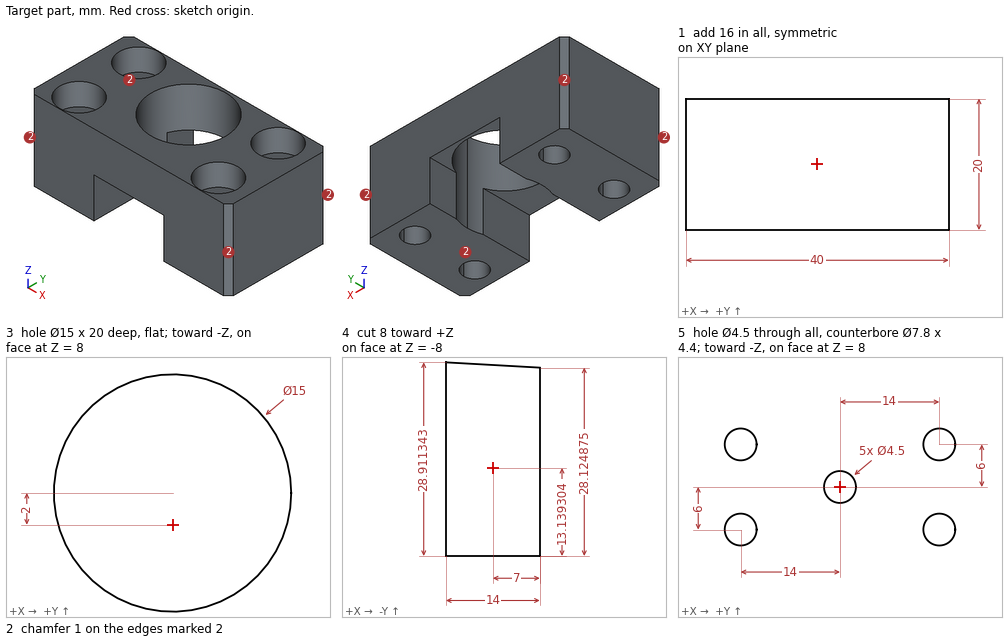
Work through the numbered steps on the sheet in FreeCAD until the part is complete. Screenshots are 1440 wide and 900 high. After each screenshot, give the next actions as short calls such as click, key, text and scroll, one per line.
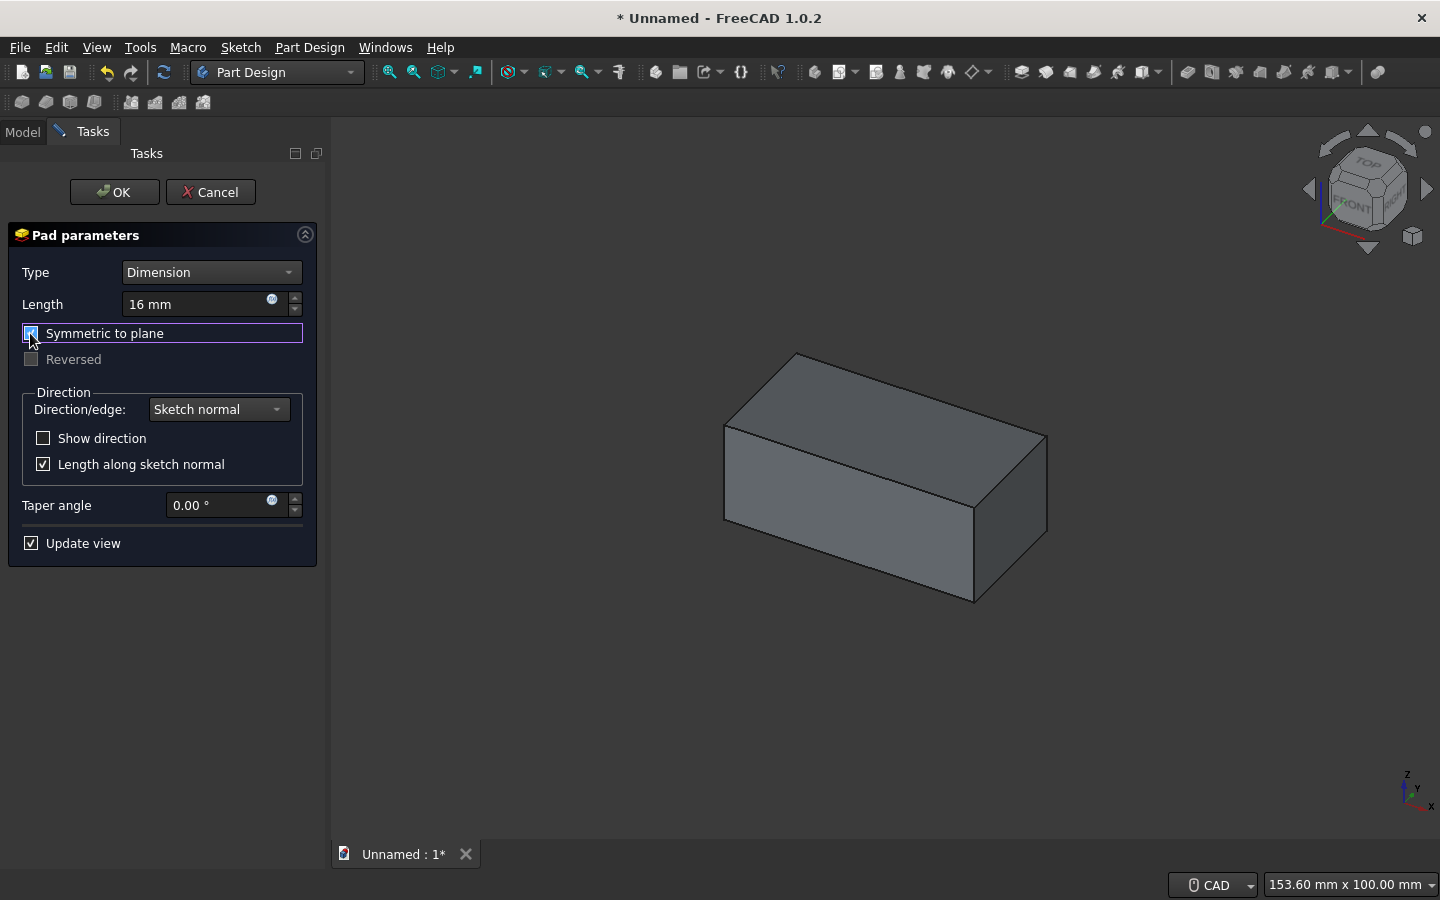
click(115, 192)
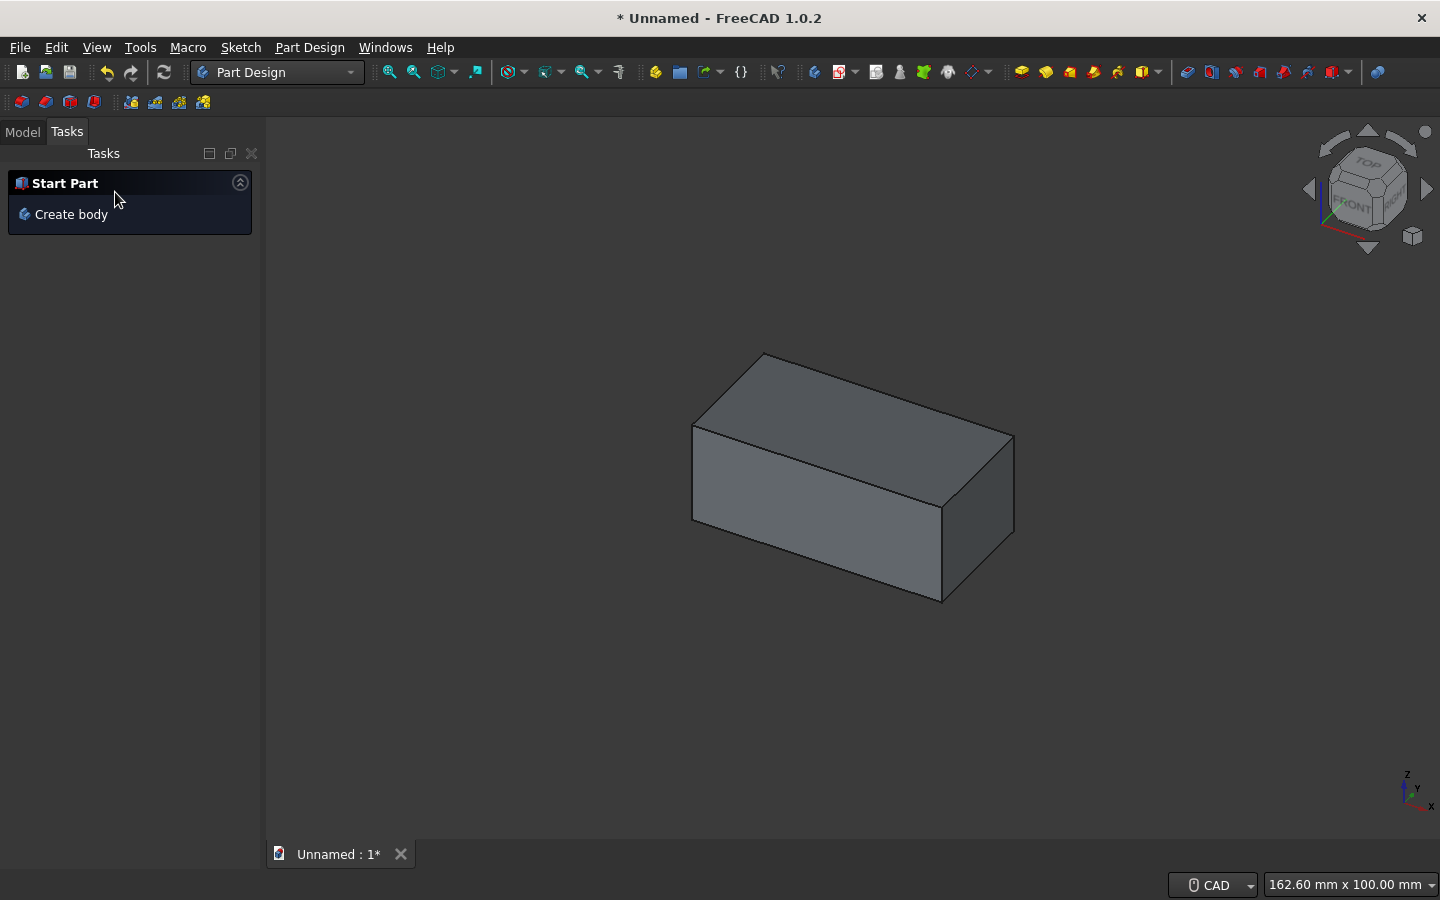
click(390, 72)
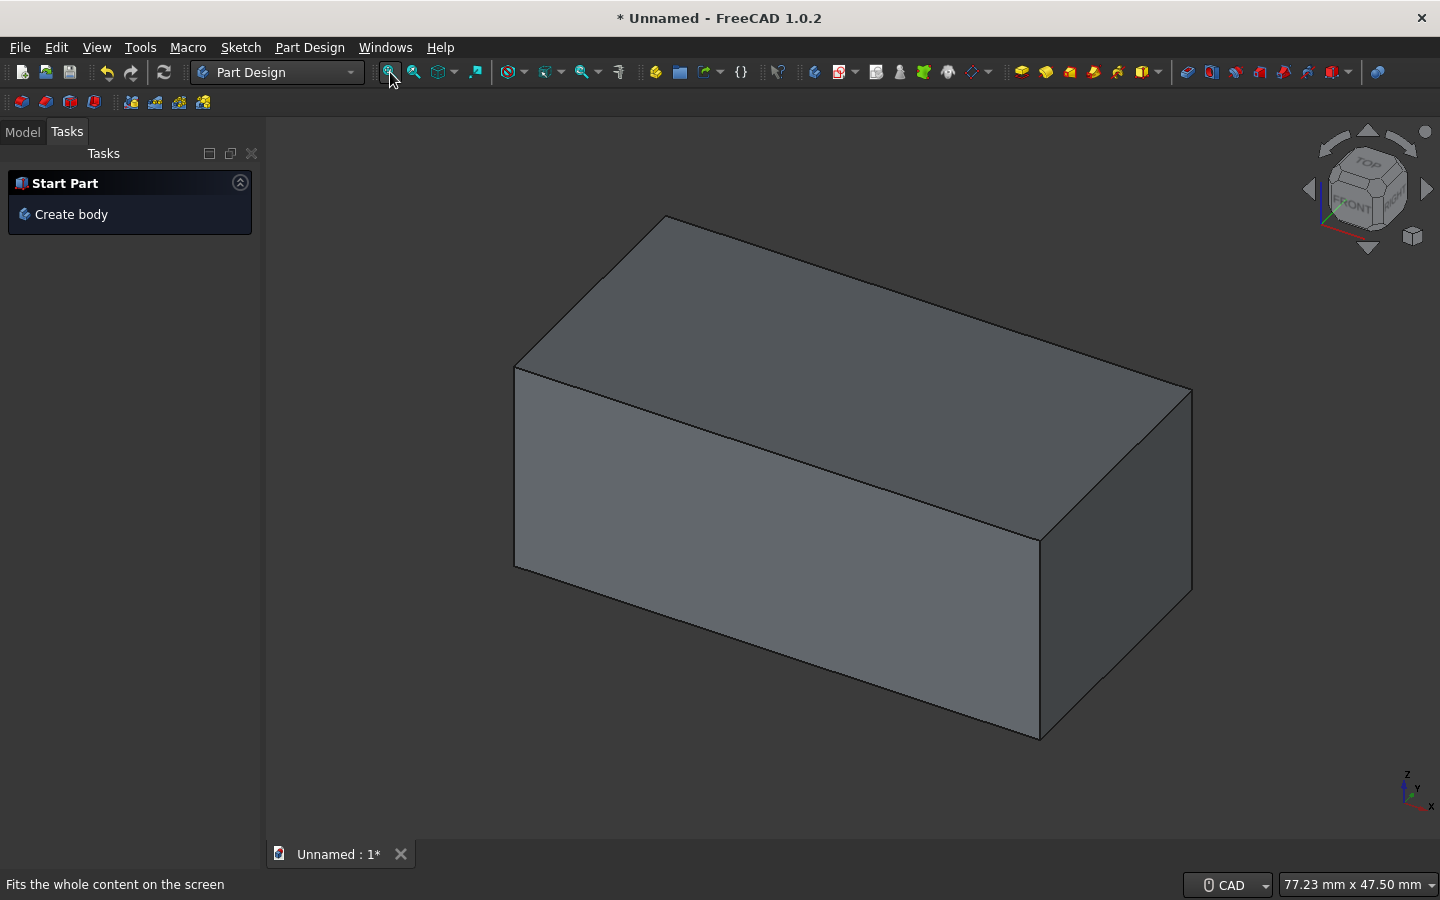
click(1040, 640)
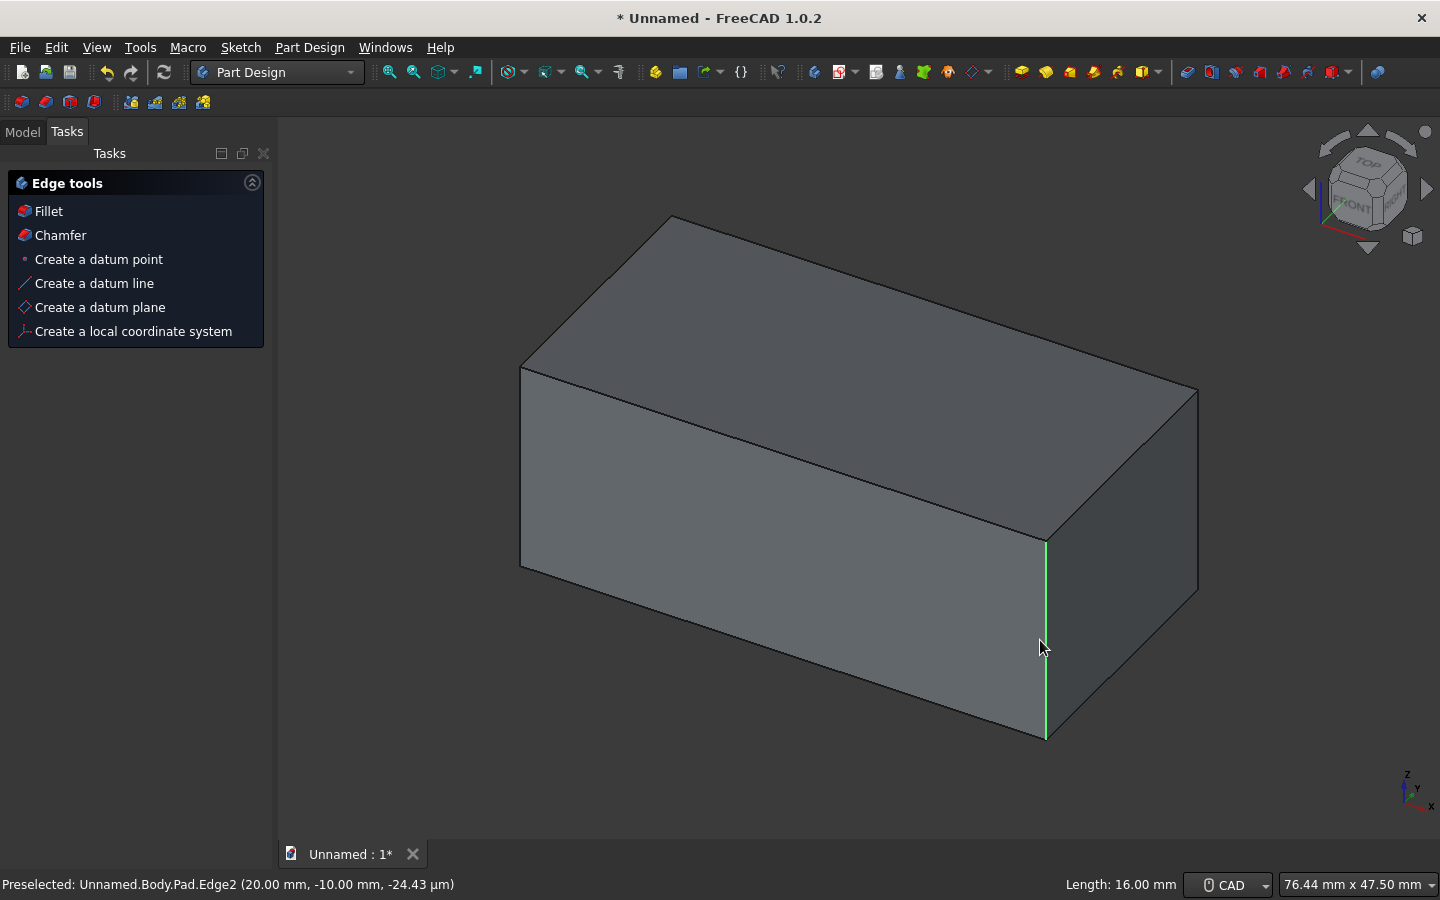
key(0)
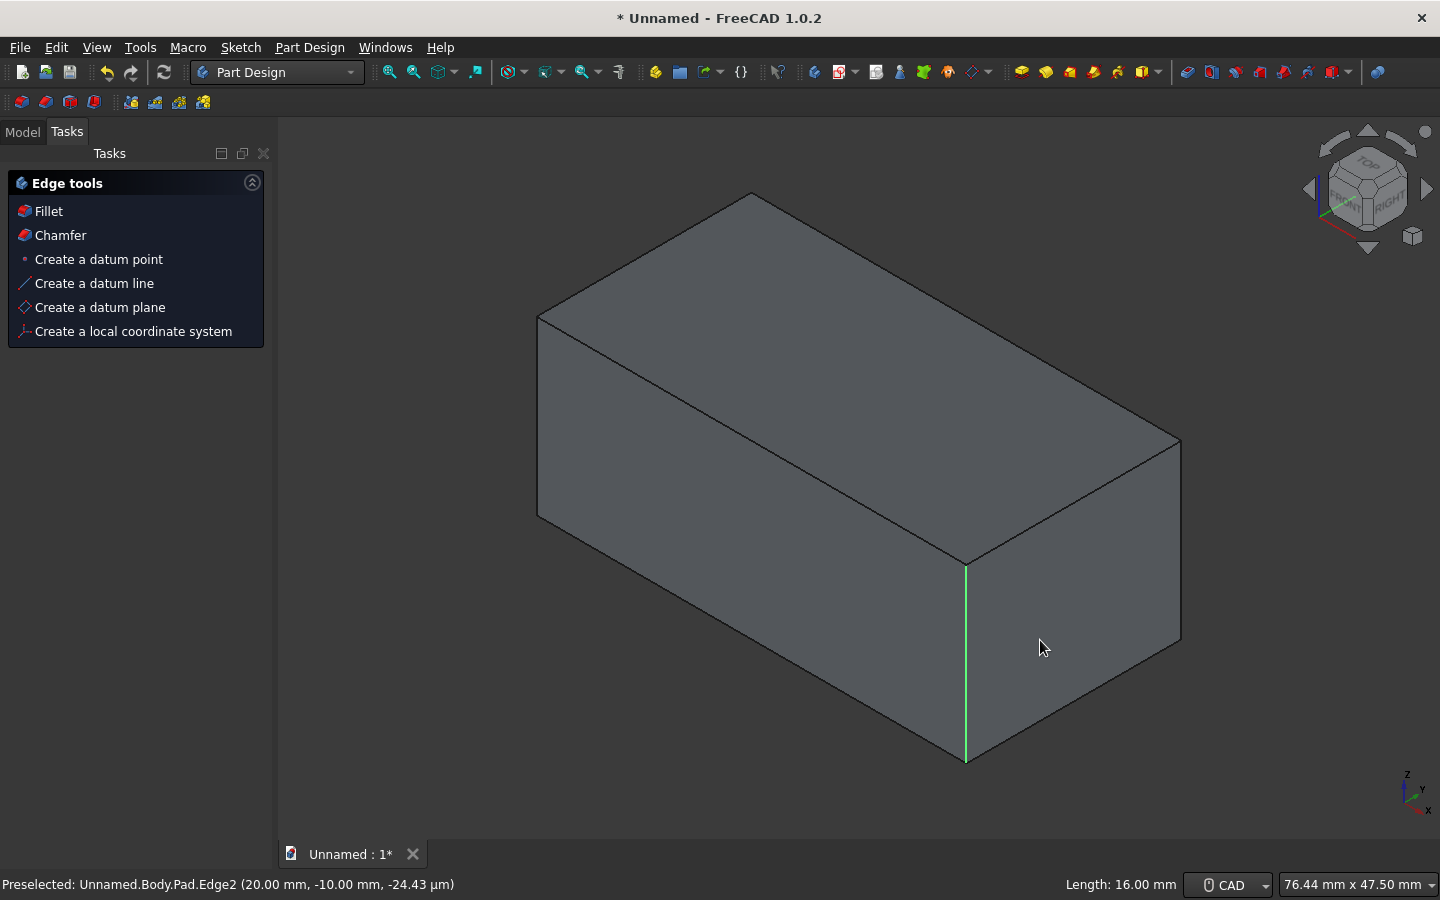
key(2)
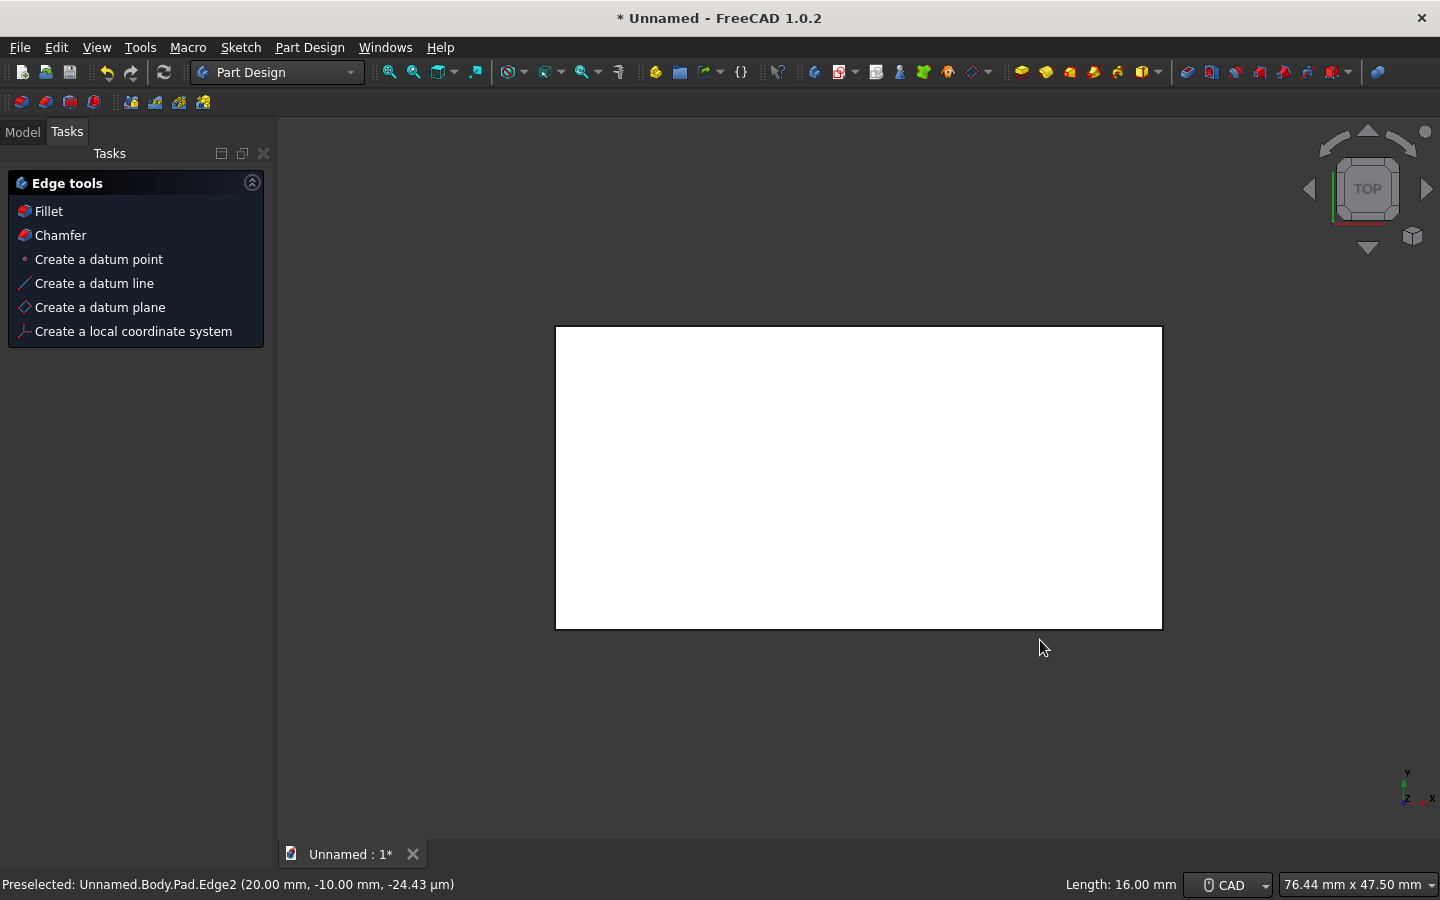
key(1)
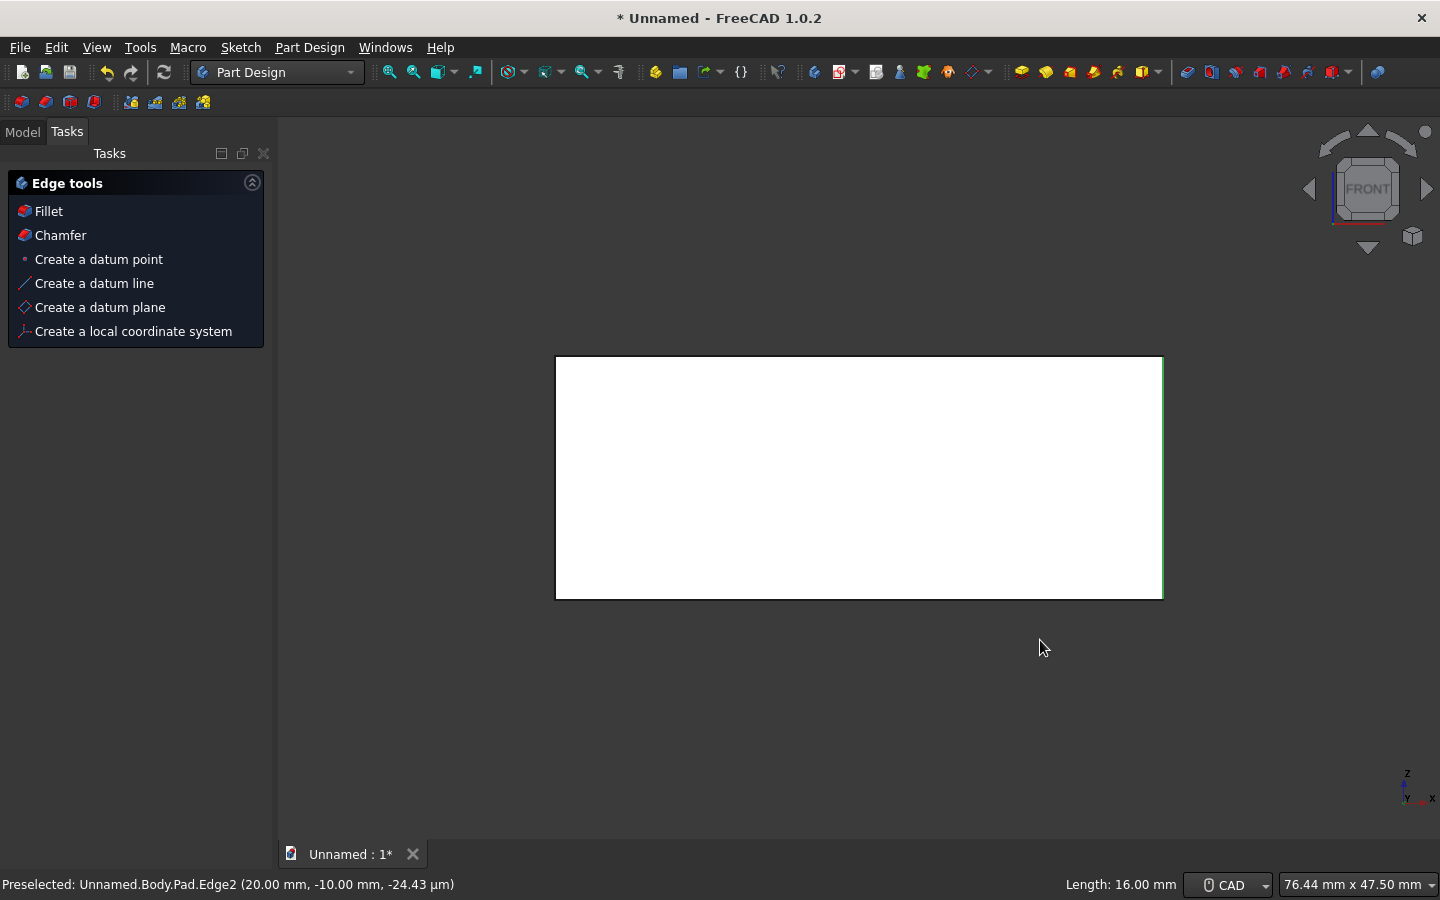
click(555, 477, ctrl)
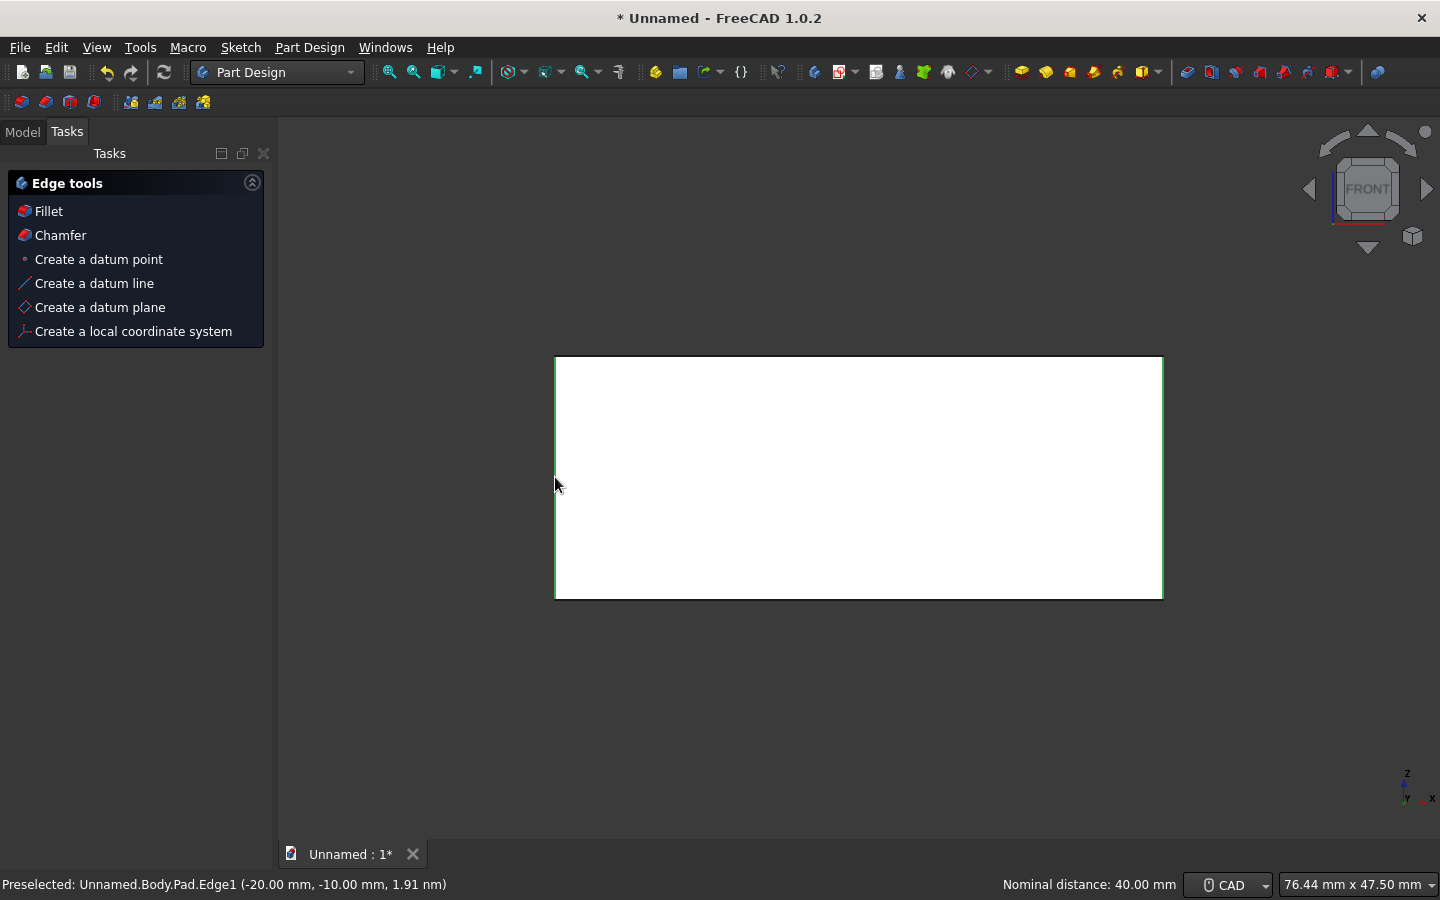
key(3)